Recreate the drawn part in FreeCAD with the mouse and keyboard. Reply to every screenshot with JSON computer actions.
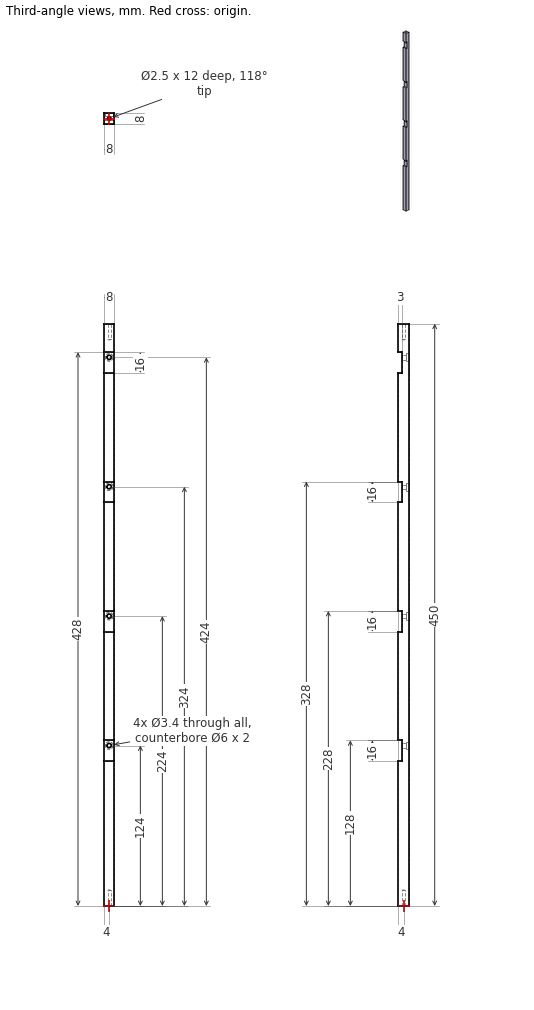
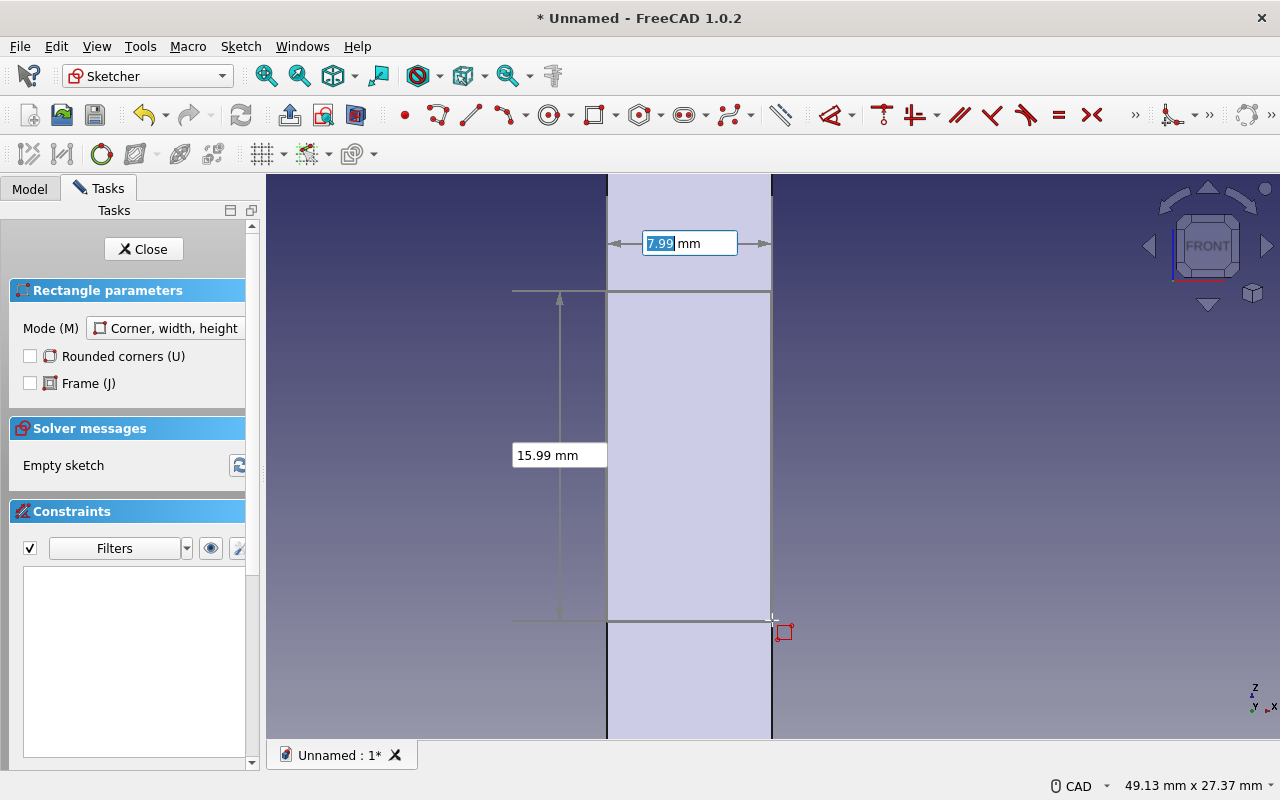
{"action": "type", "text": "8"}
{"action": "key", "text": "Tab"}
{"action": "type", "text": "16"}
{"action": "key", "text": "Return"}
{"action": "key", "text": "Escape"}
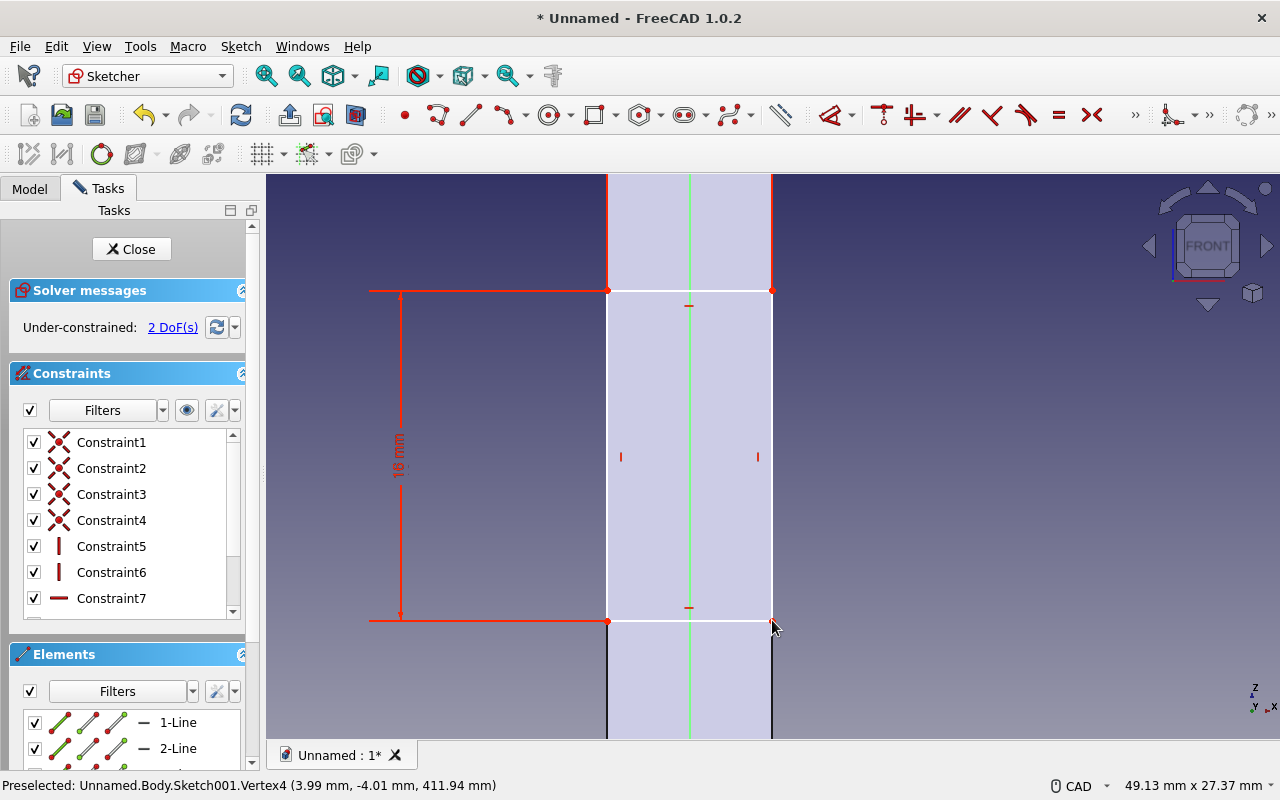
{"action": "left_click", "coordinate": [830, 116]}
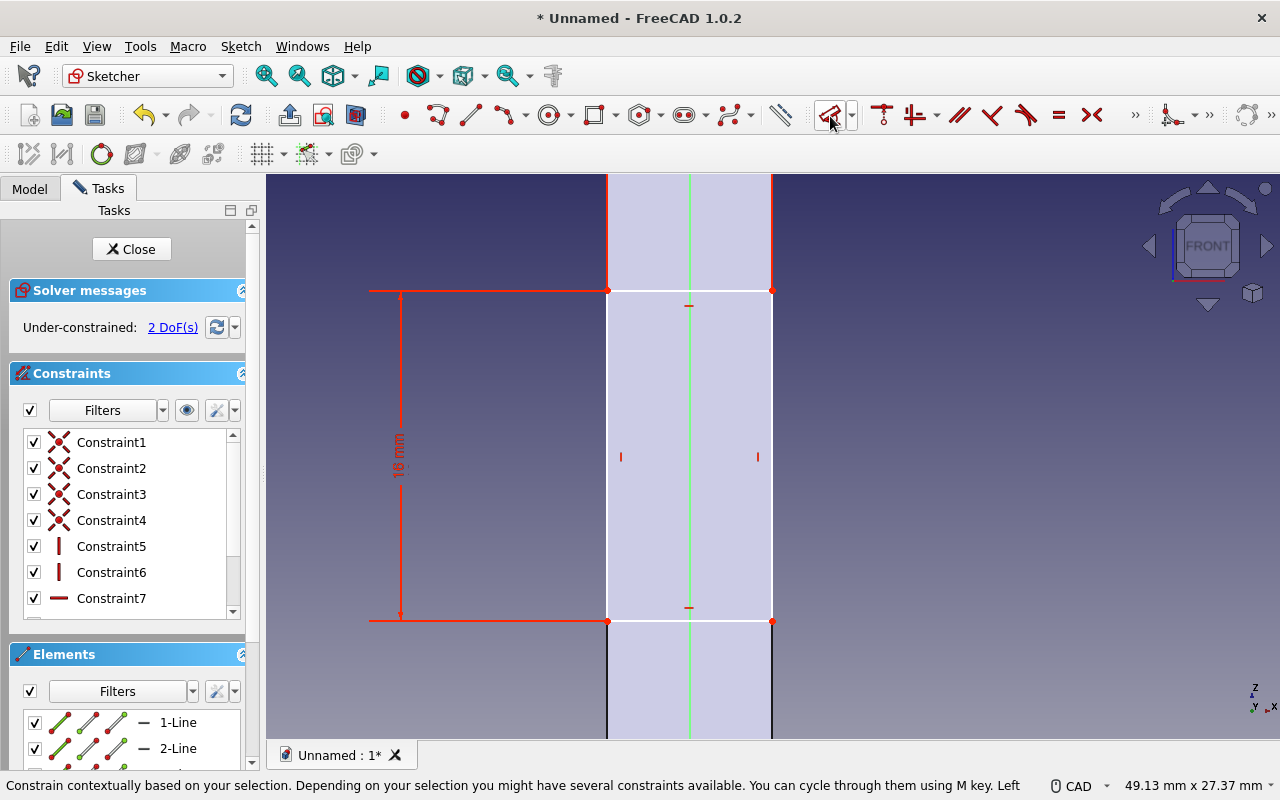
{"action": "left_click", "coordinate": [607, 291]}
{"action": "left_click", "coordinate": [648, 257]}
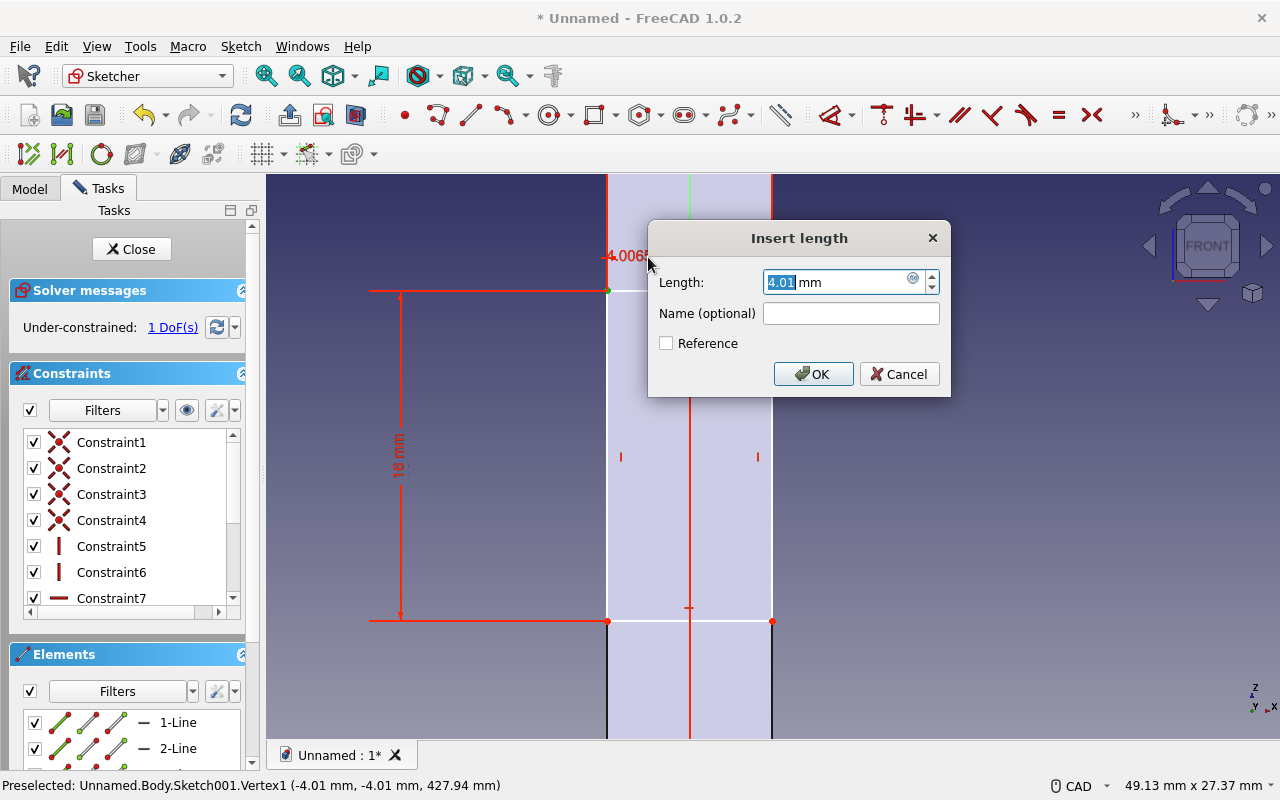
{"action": "type", "text": "4"}
{"action": "key", "text": "Return"}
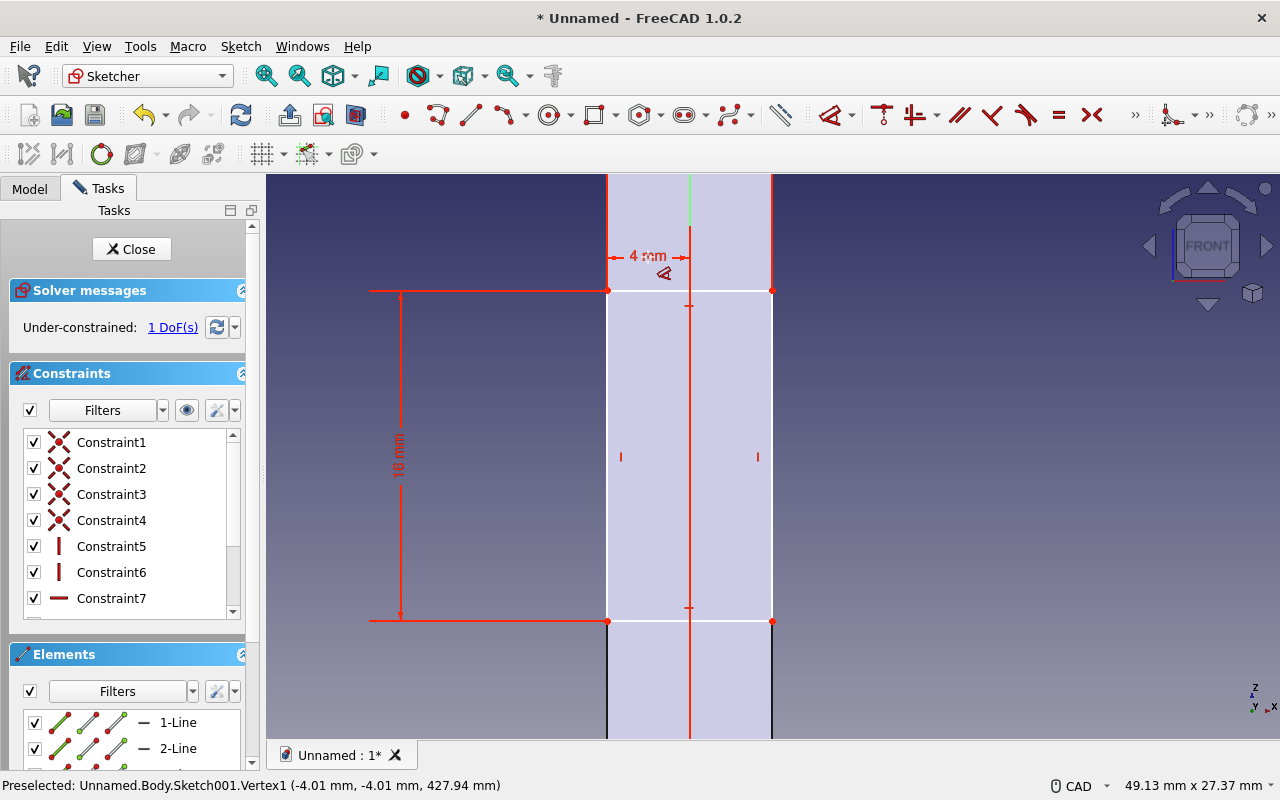
{"action": "left_click", "coordinate": [607, 291]}
{"action": "left_click", "coordinate": [573, 501]}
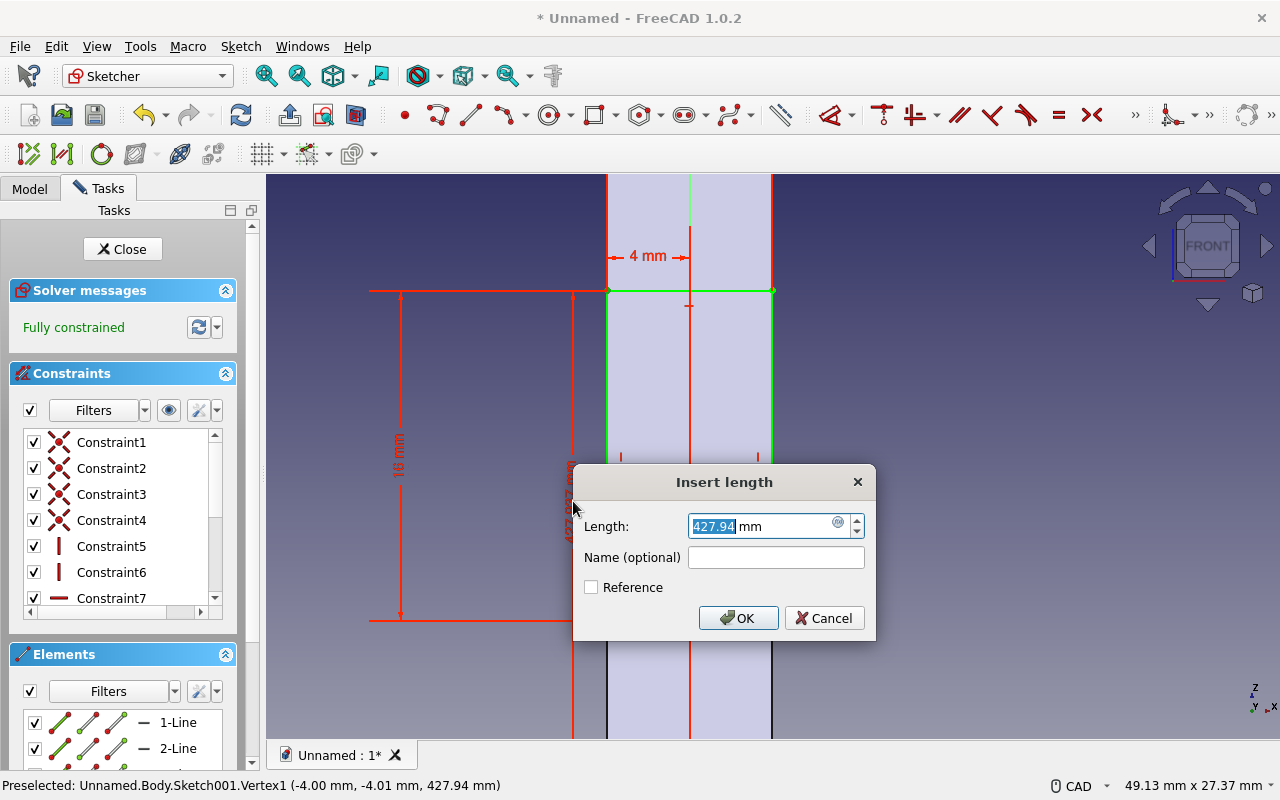
{"action": "type", "text": "428"}
{"action": "key", "text": "Return"}
{"action": "key", "text": "Escape"}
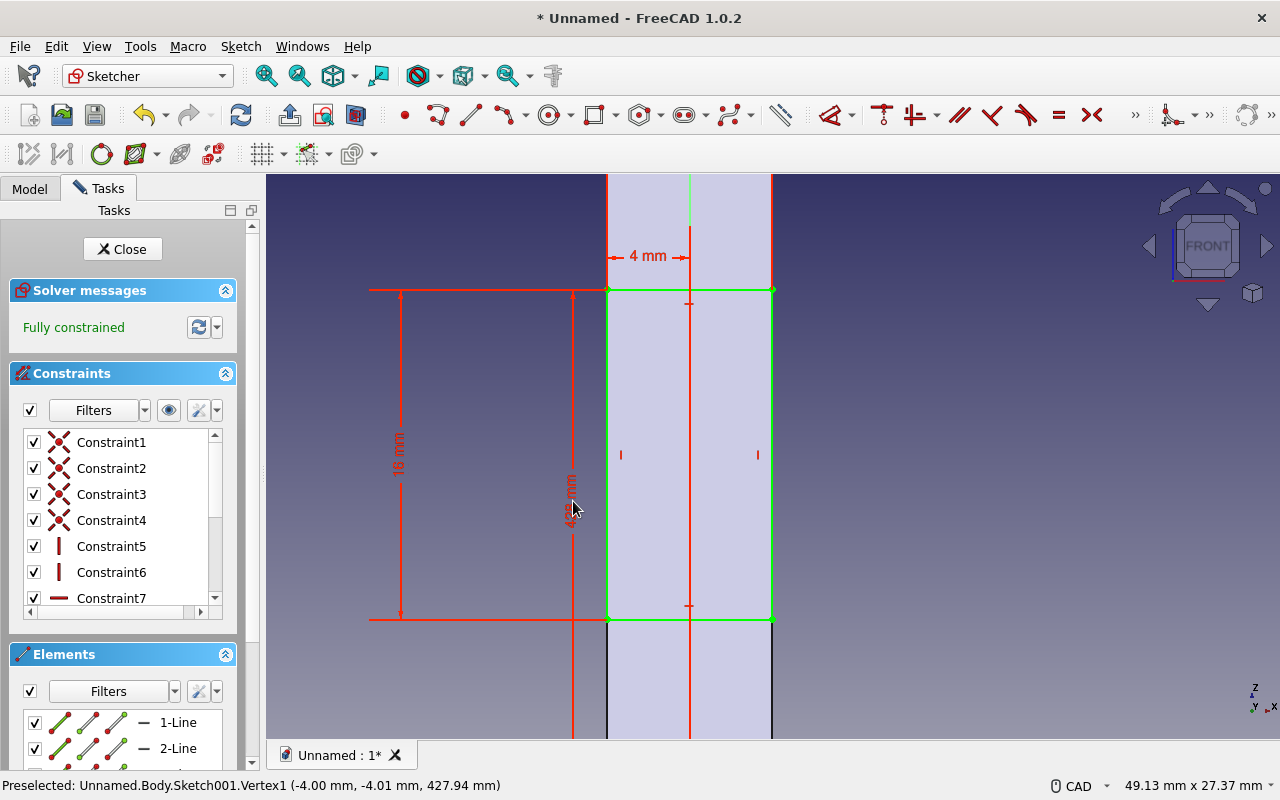
{"action": "left_click", "coordinate": [123, 249]}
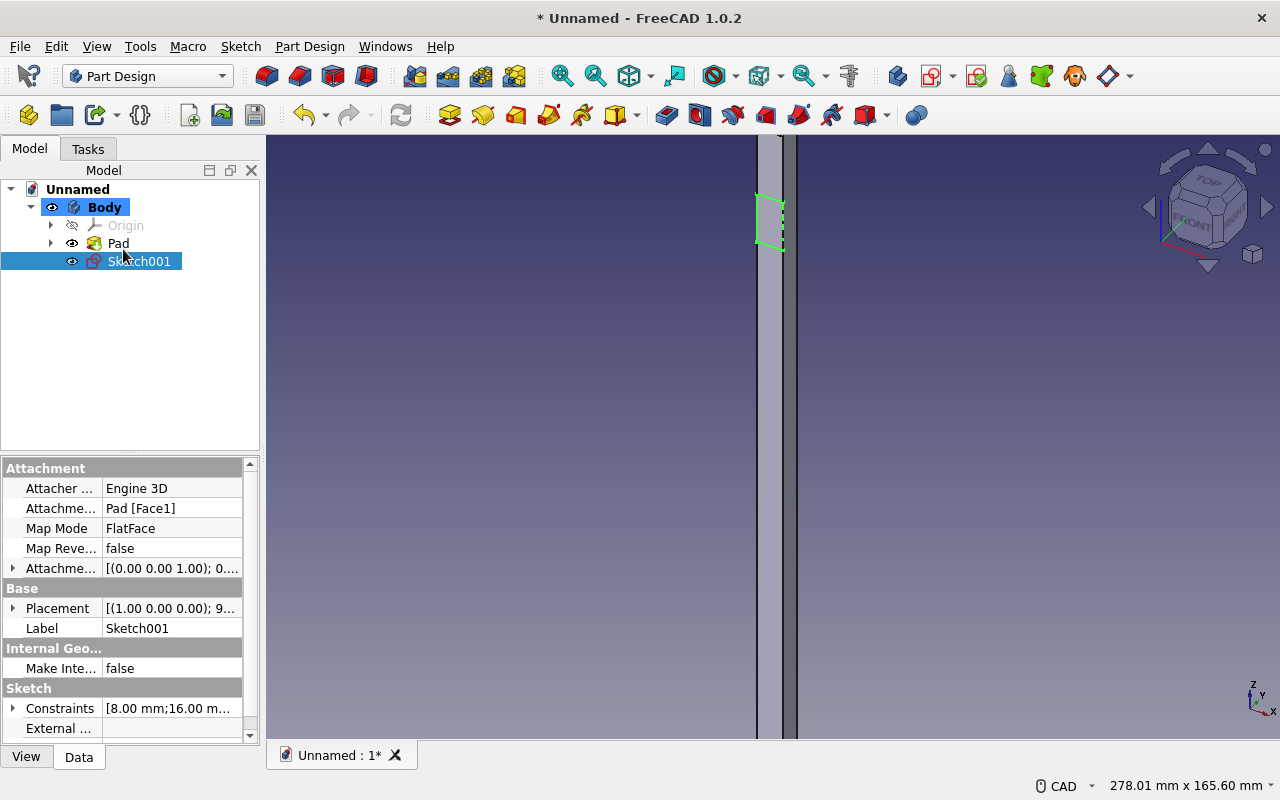
{"action": "left_click", "coordinate": [667, 116]}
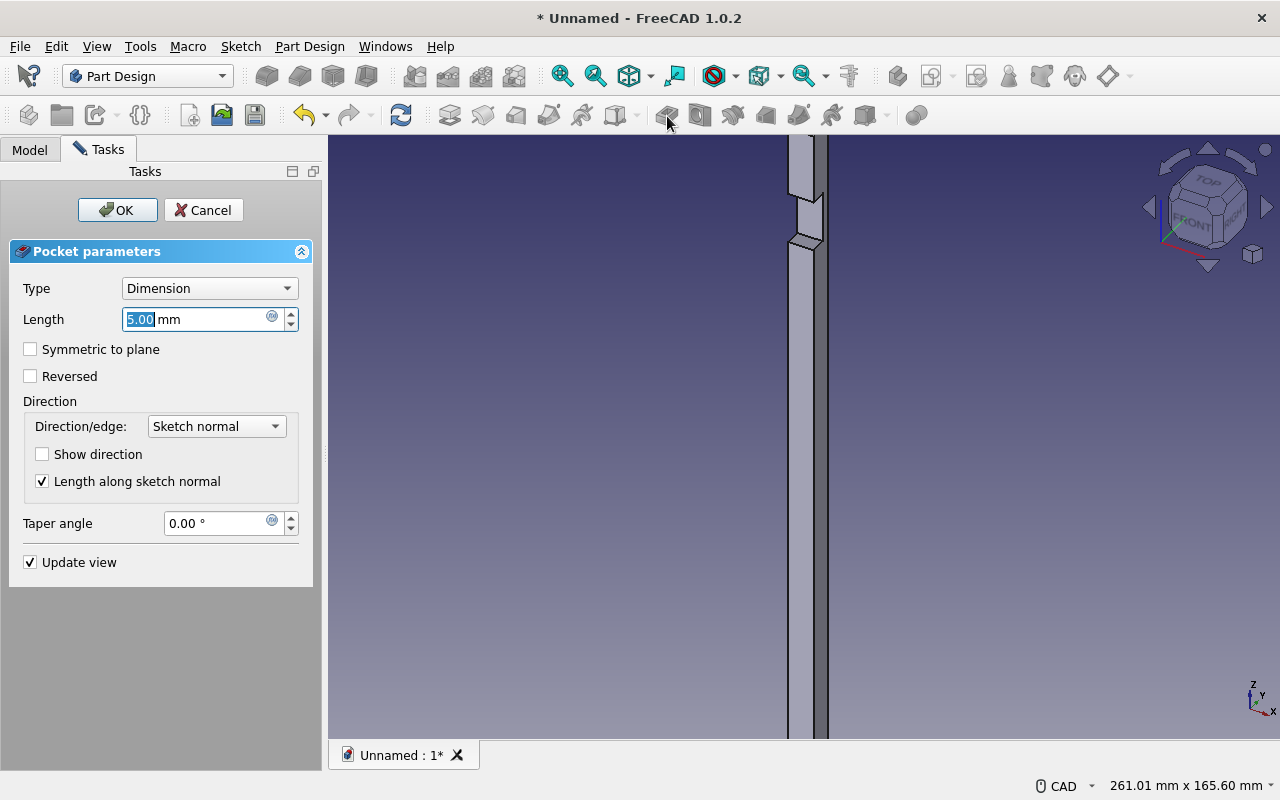
{"action": "type", "text": "3"}
{"action": "key", "text": "Tab"}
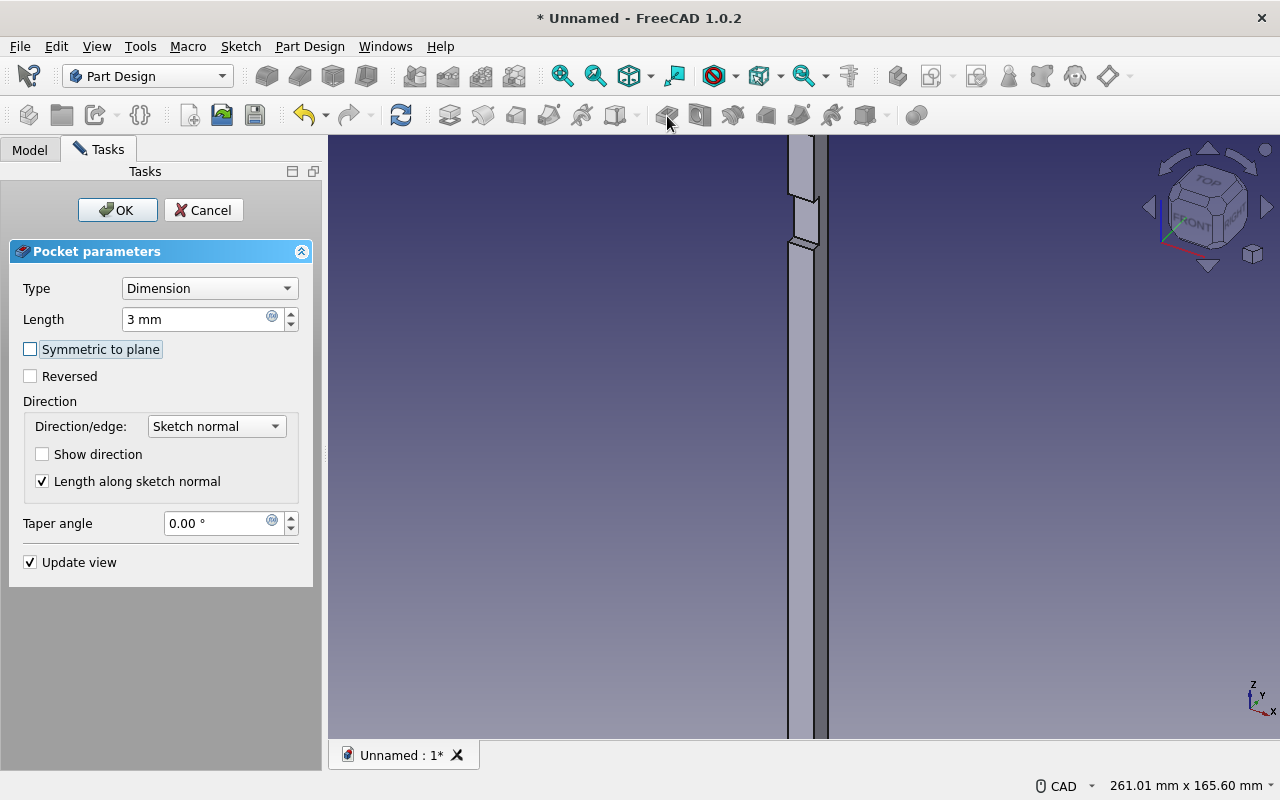
{"action": "left_click", "coordinate": [118, 210]}